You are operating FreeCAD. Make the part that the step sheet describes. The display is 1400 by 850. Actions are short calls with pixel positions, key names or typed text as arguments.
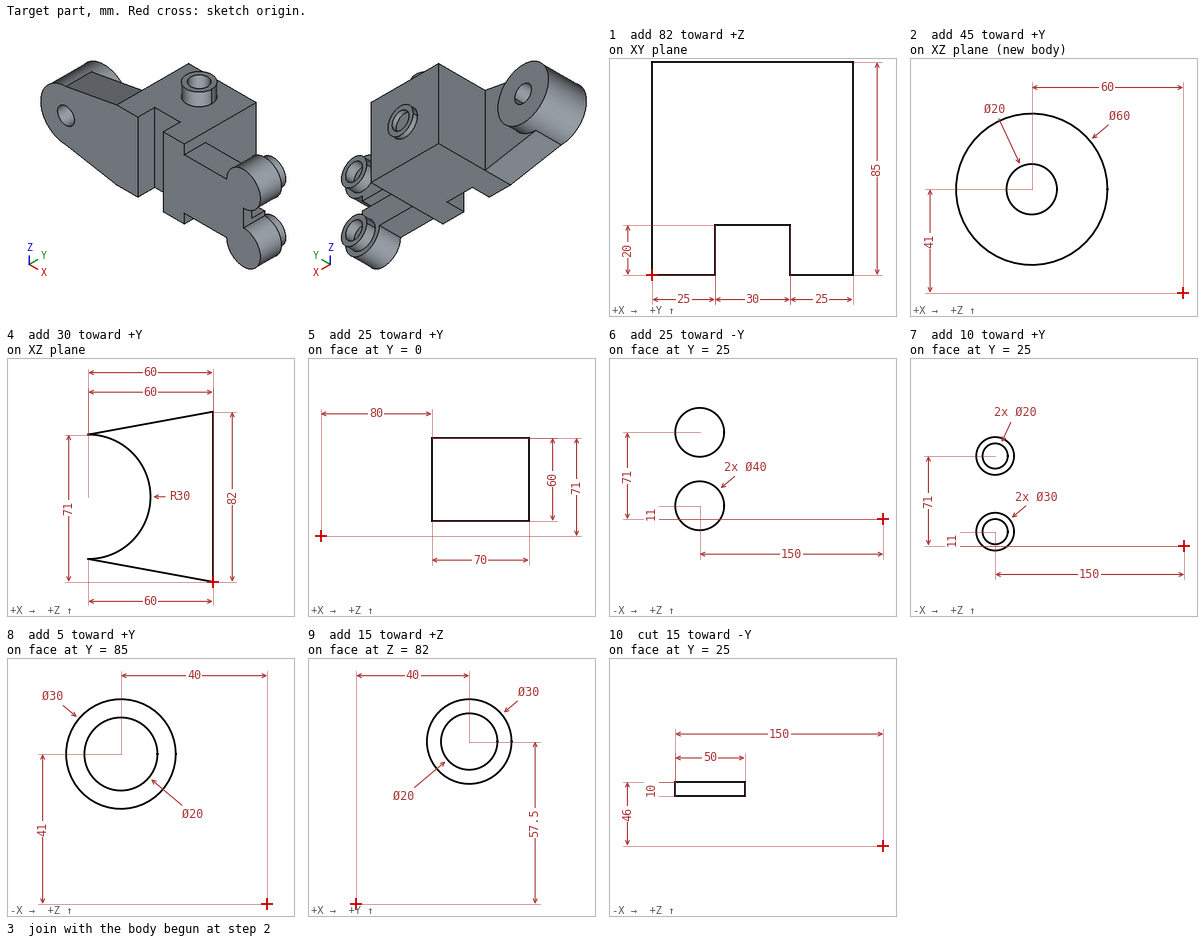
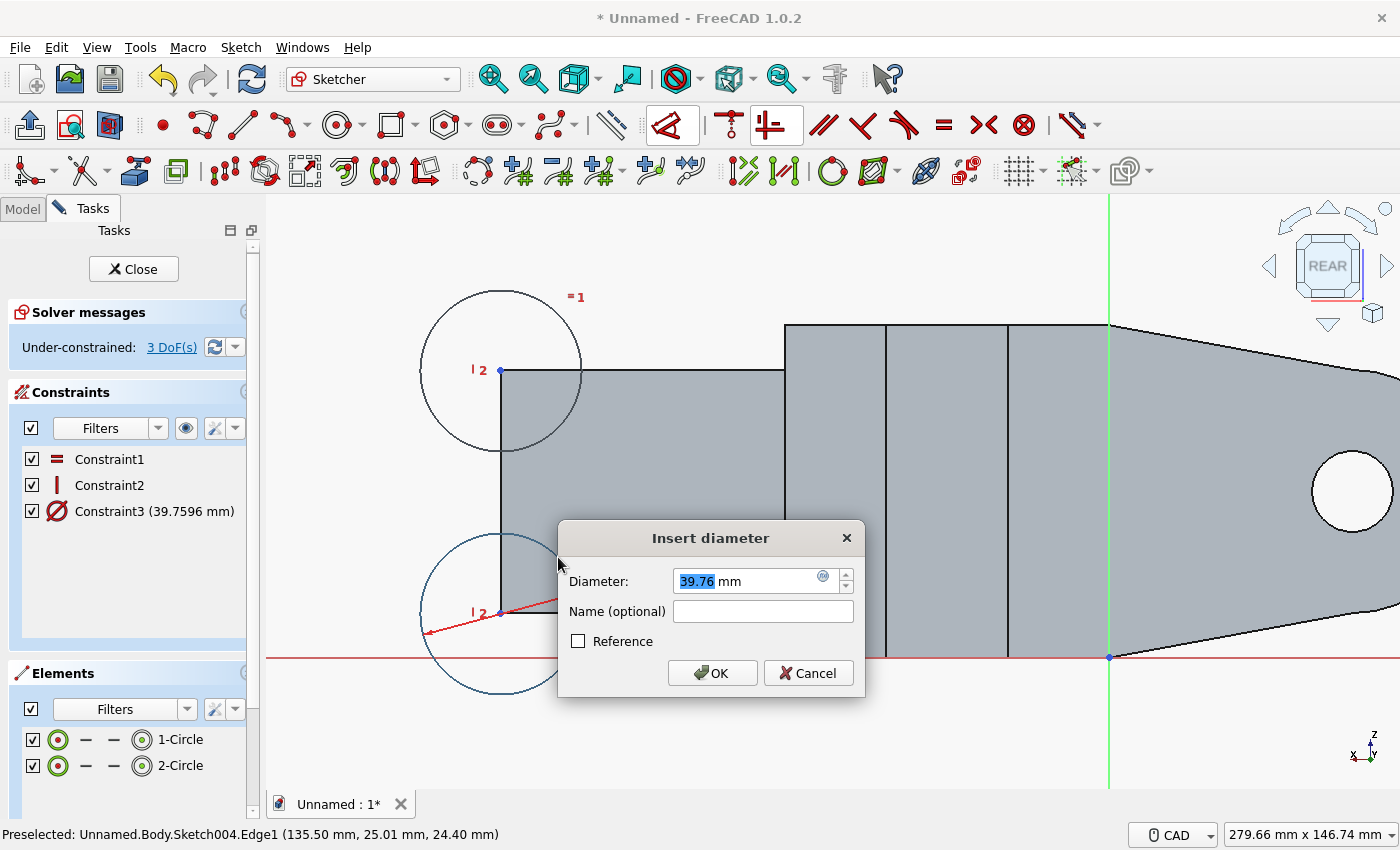
text(40)
key(Return)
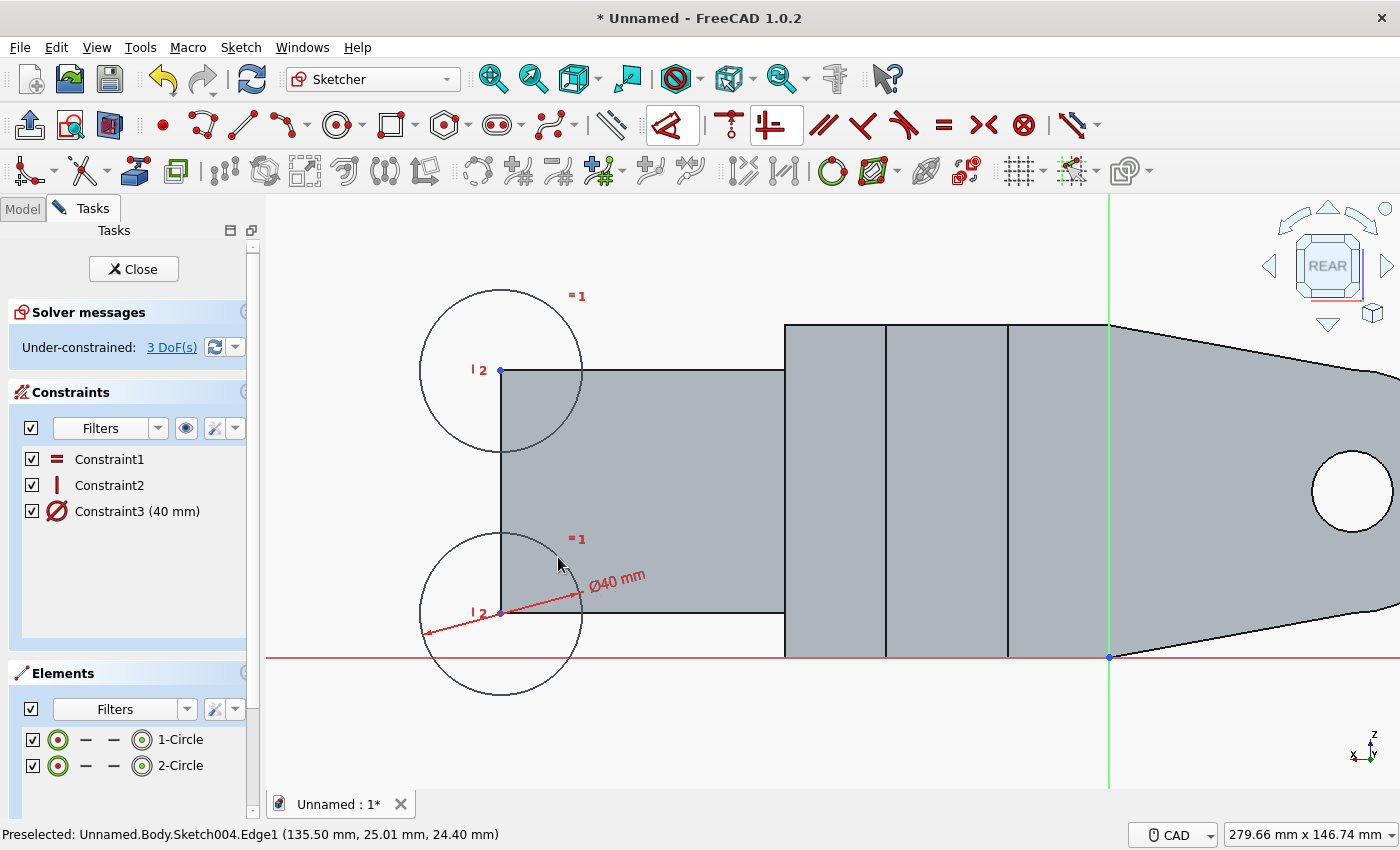
click(501, 614)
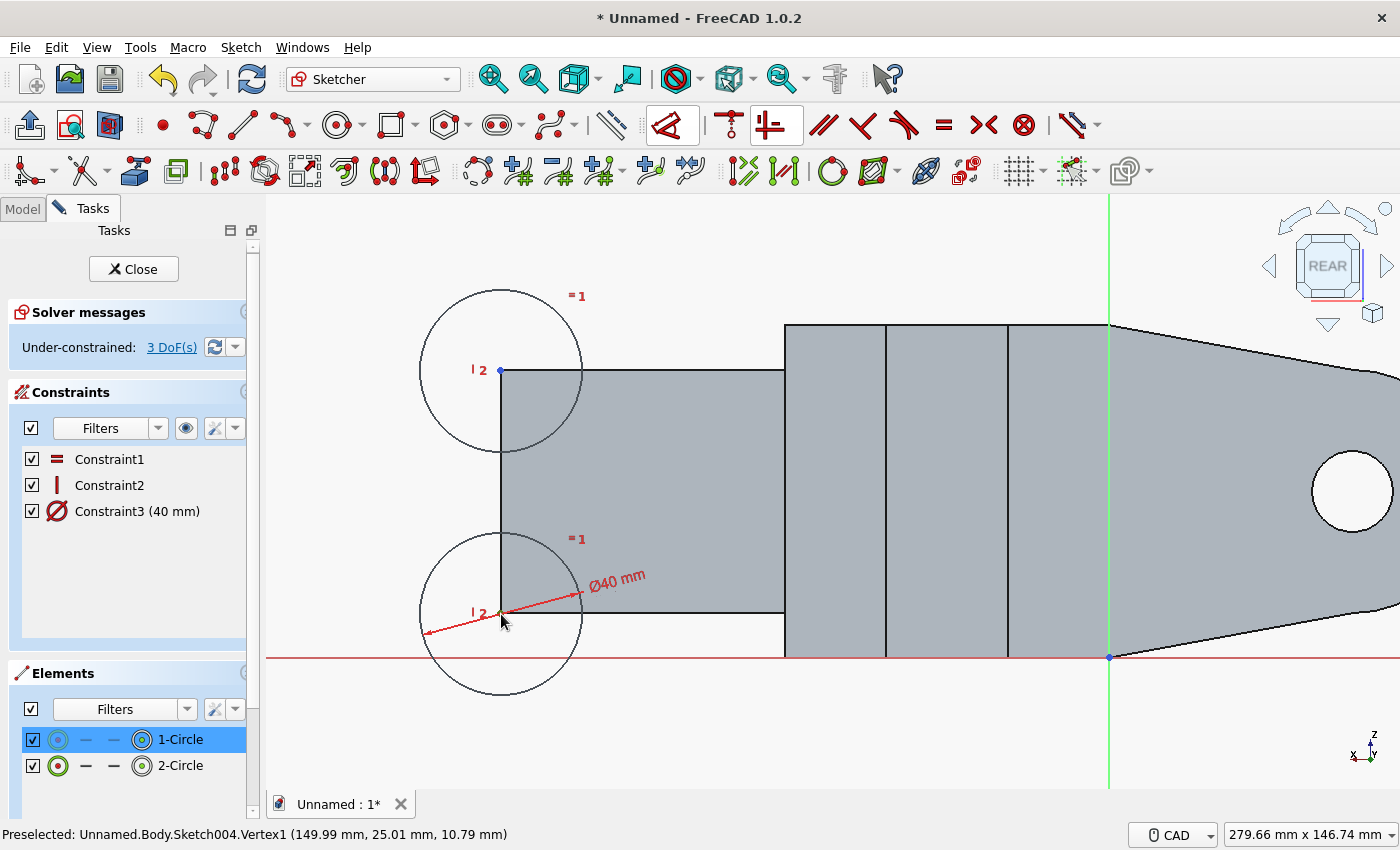
click(694, 126)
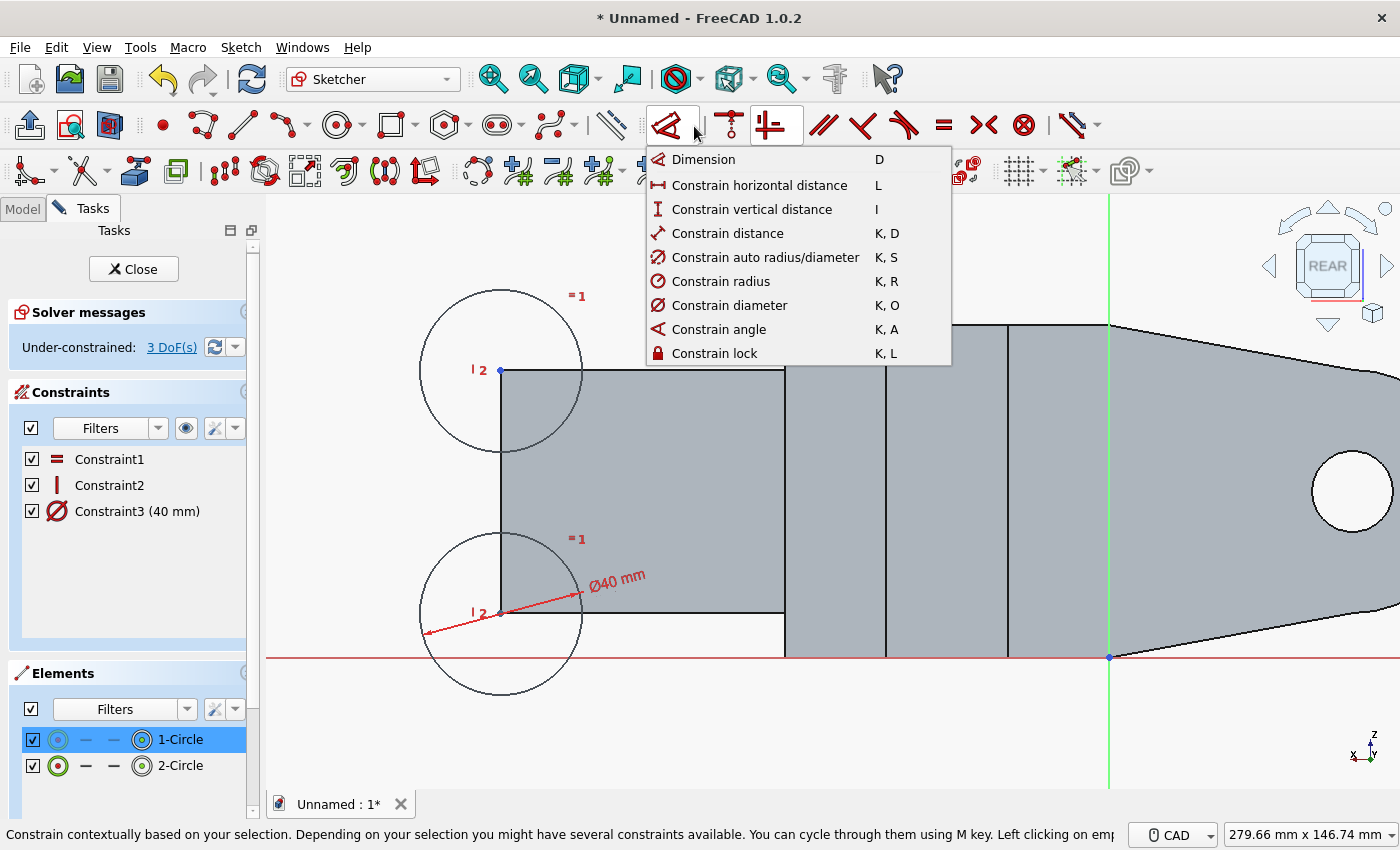
click(799, 209)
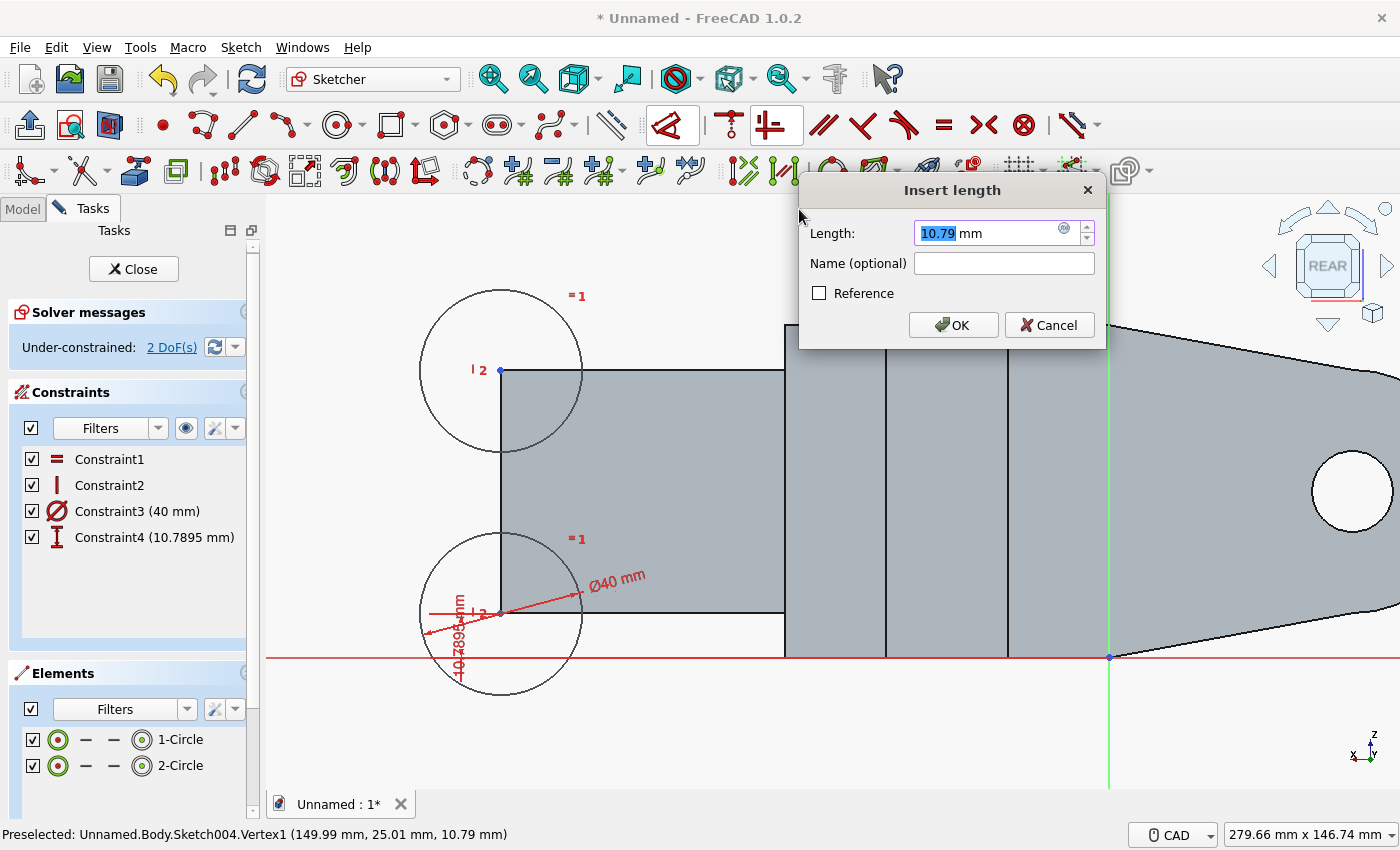
text(11)
key(Return)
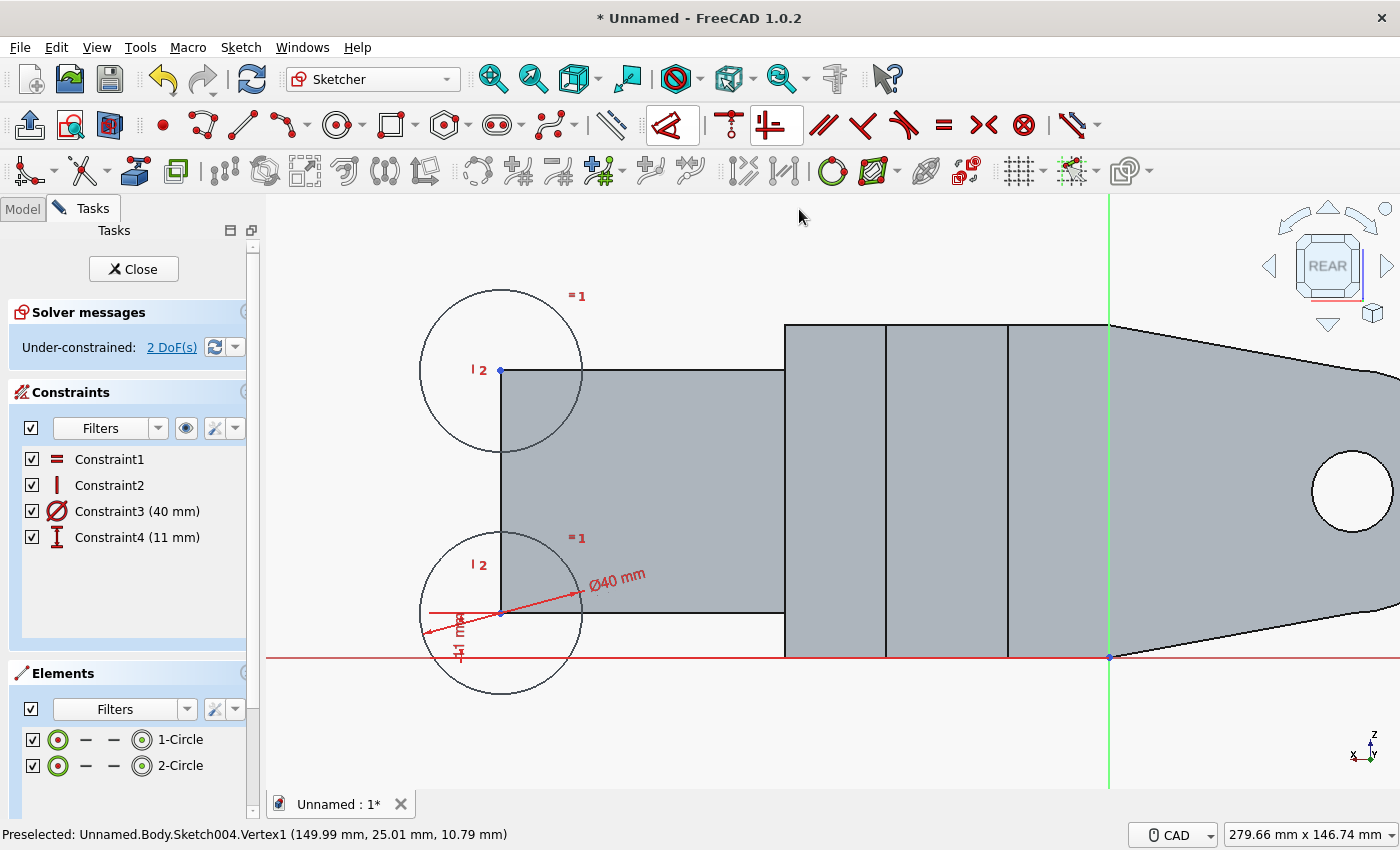
click(501, 371)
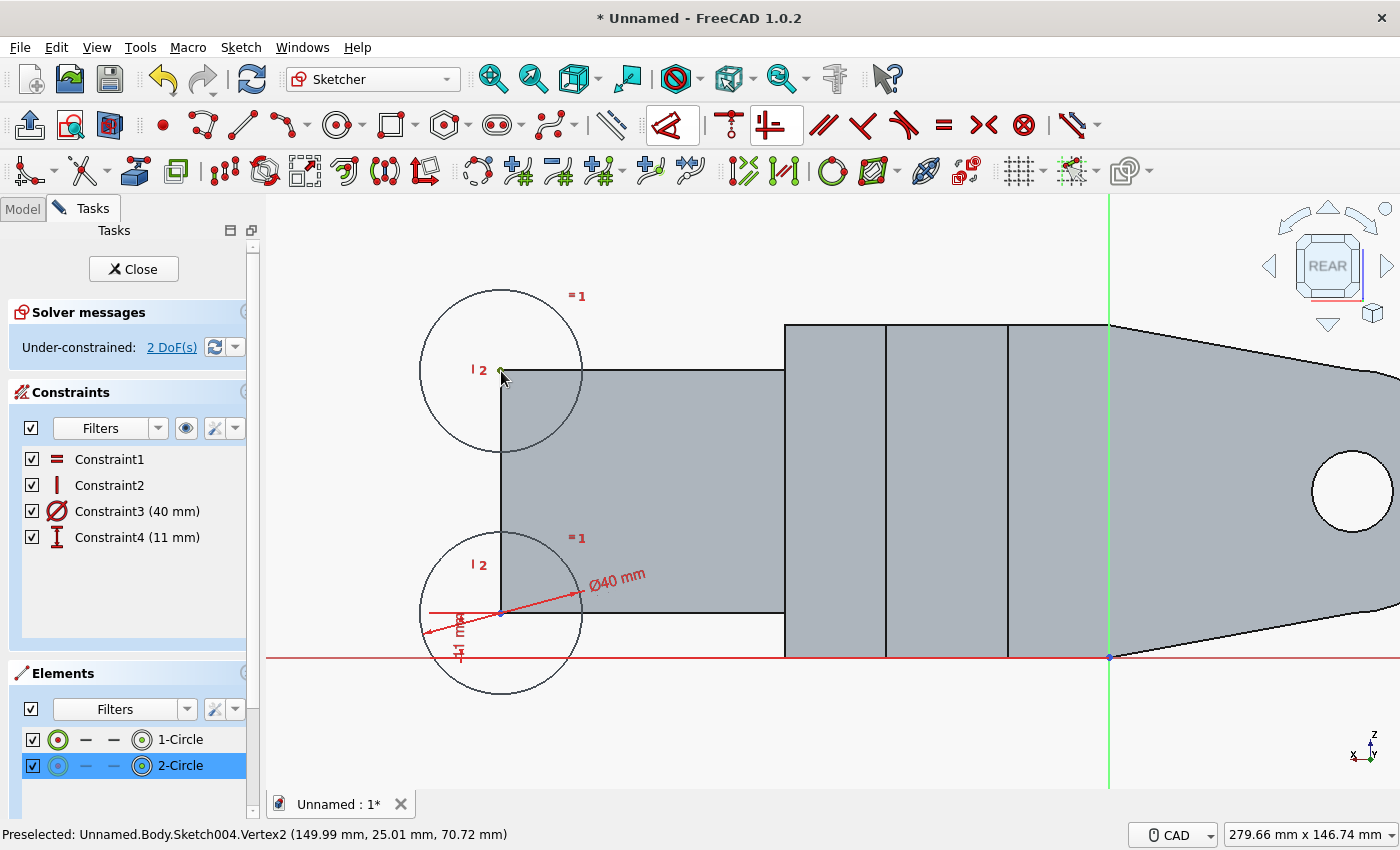
key(i)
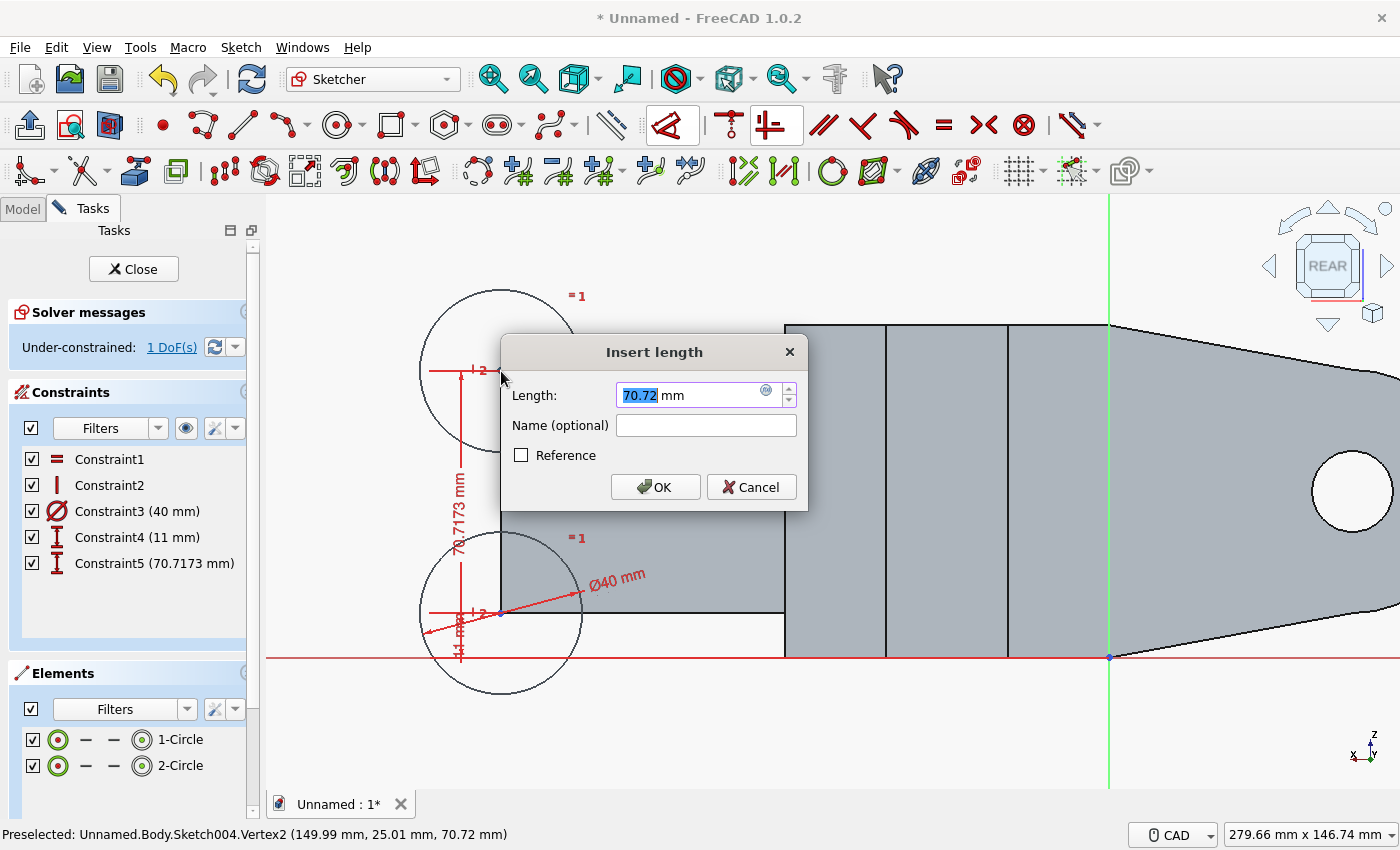
text(71)
key(Return)